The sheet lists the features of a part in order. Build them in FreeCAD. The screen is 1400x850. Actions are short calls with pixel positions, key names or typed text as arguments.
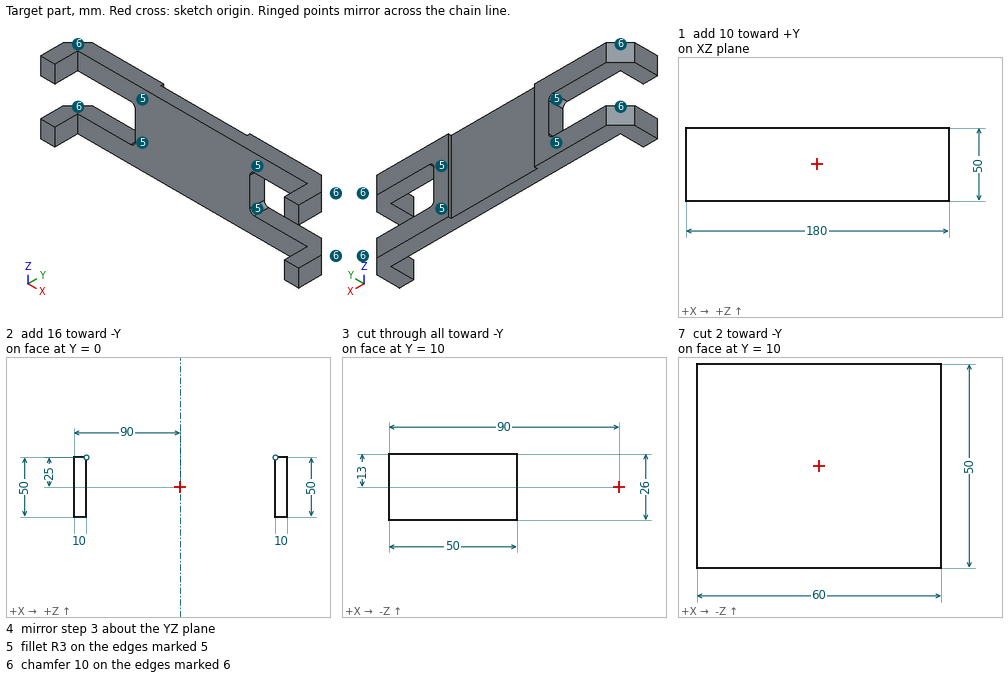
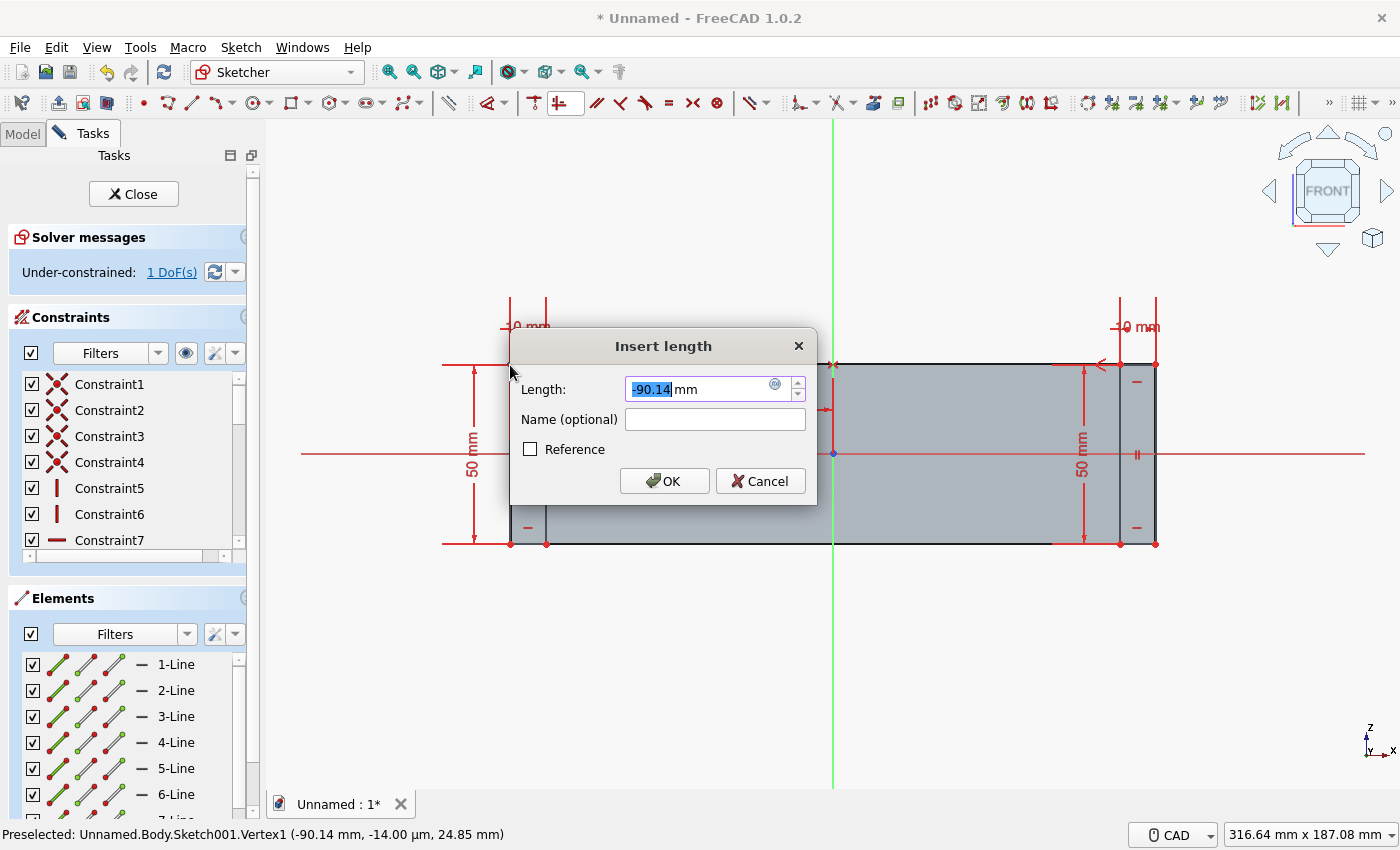
text(-90)
key(Return)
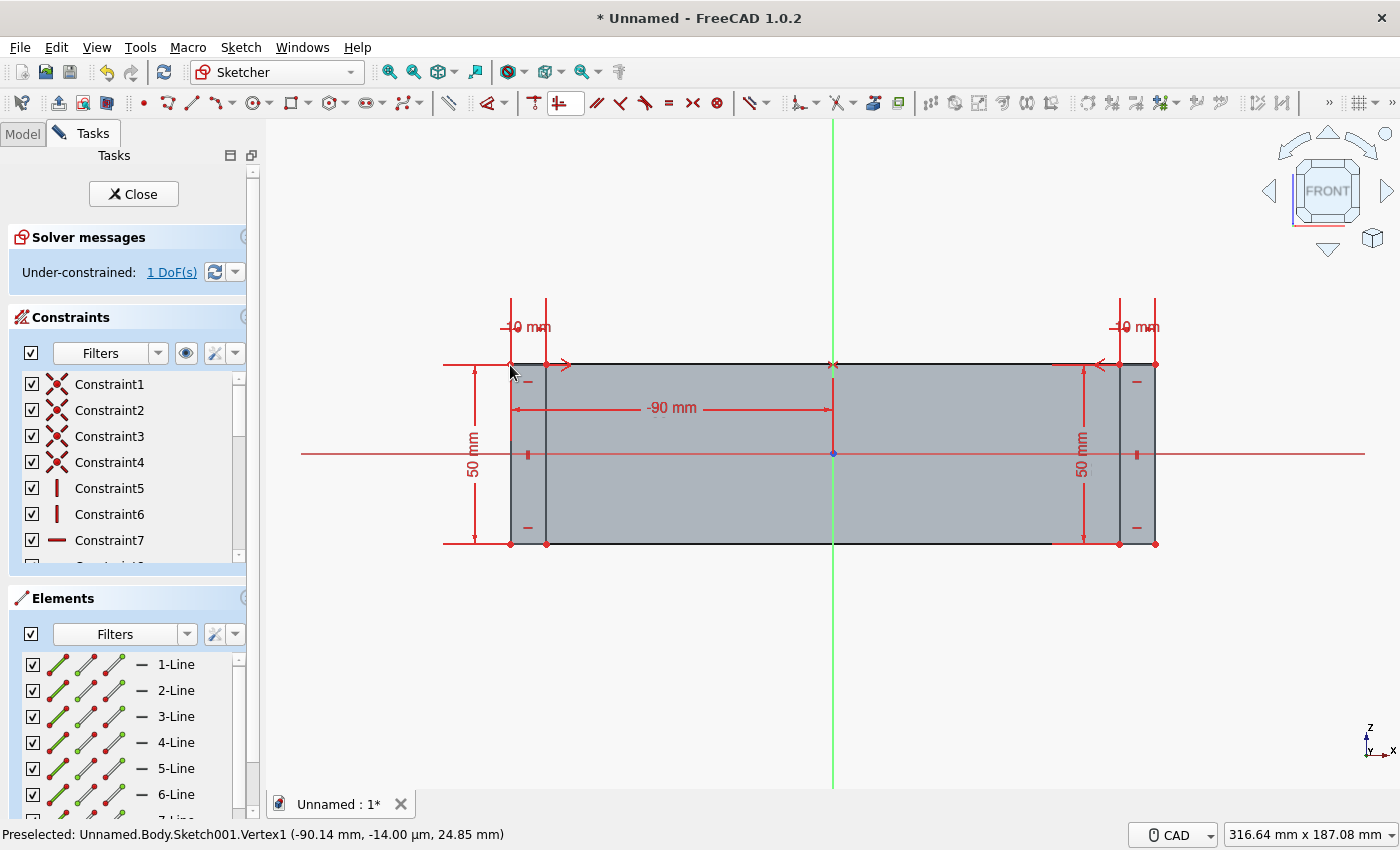
click(511, 365)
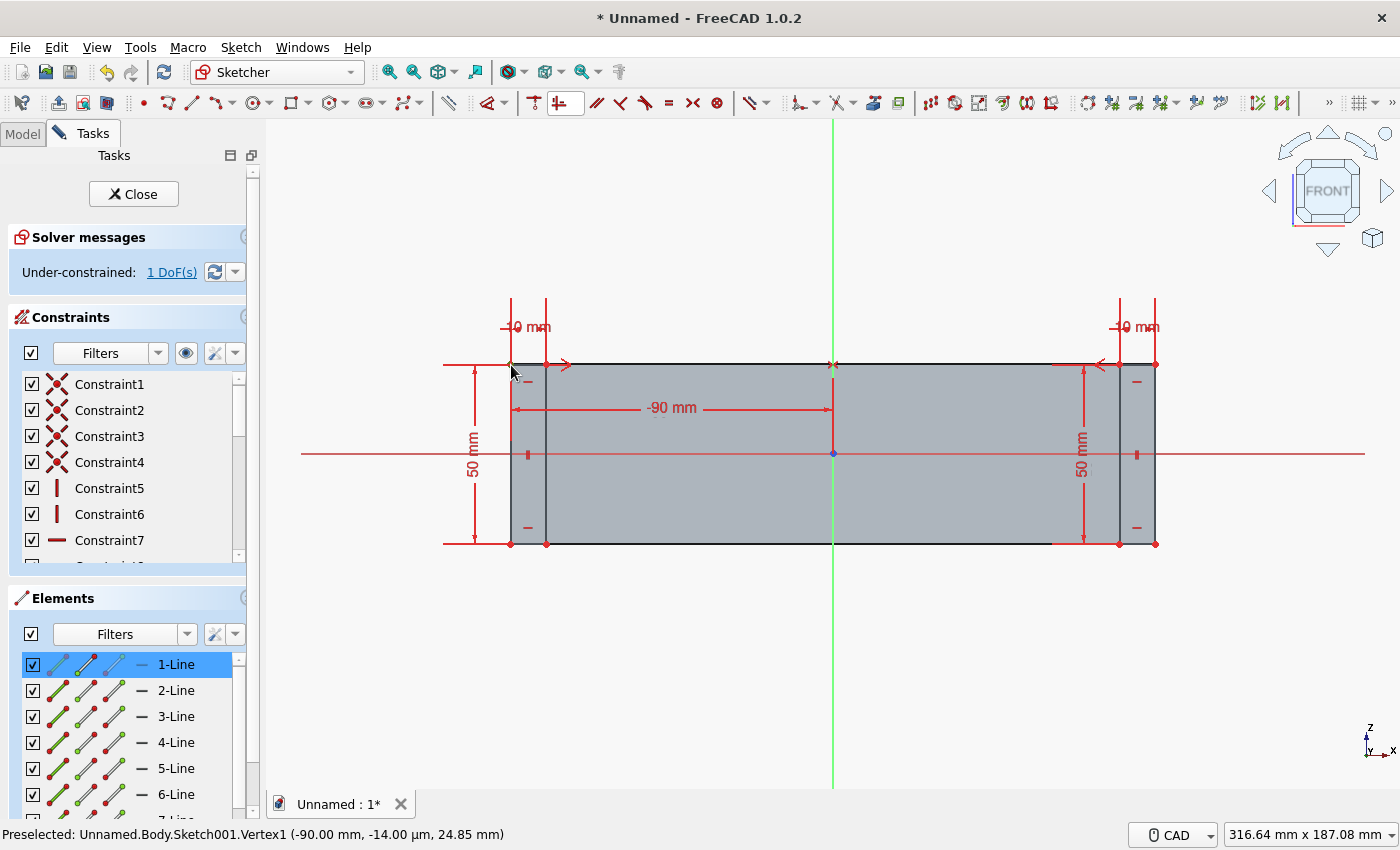
key(i)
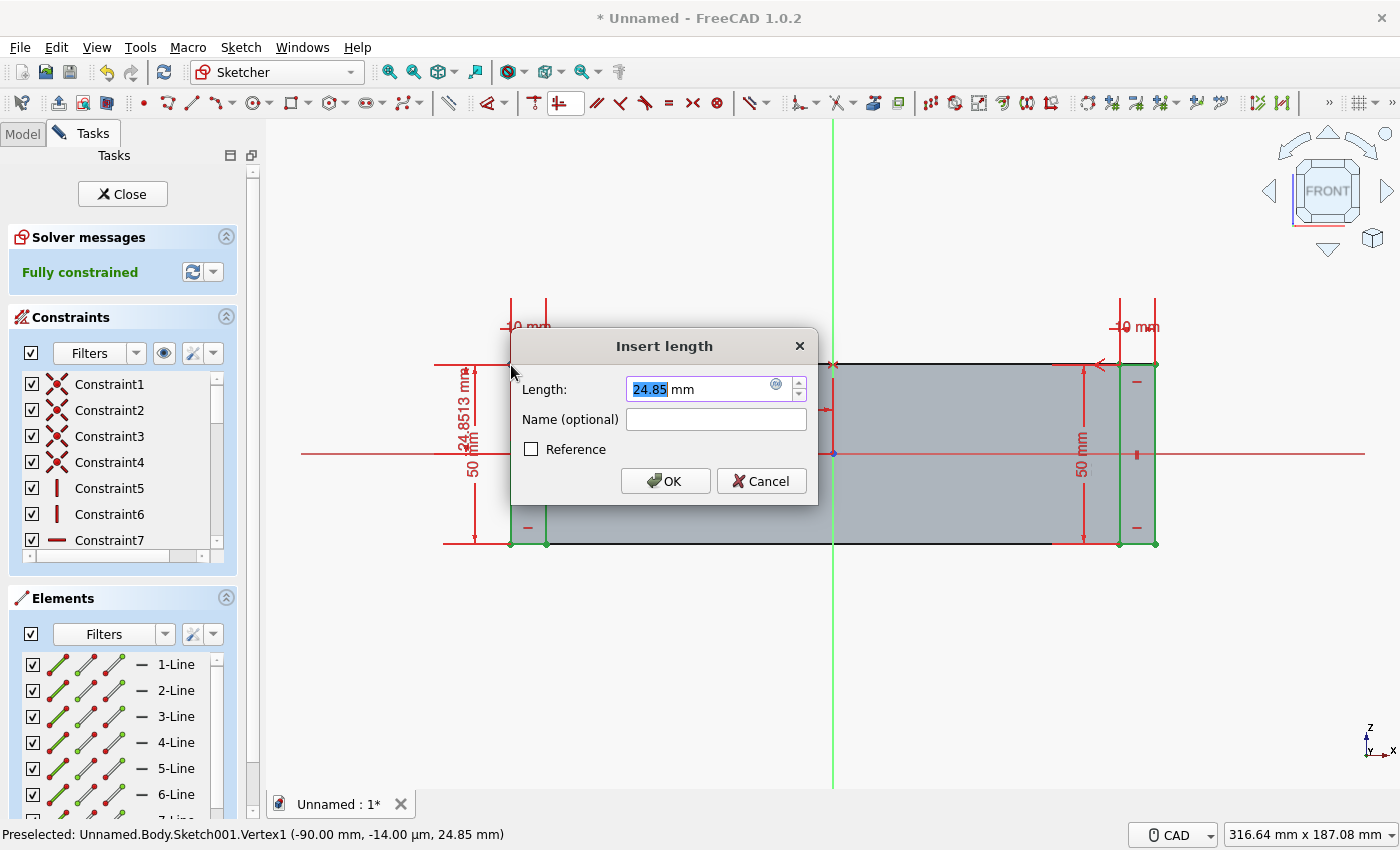
text(25)
key(Return)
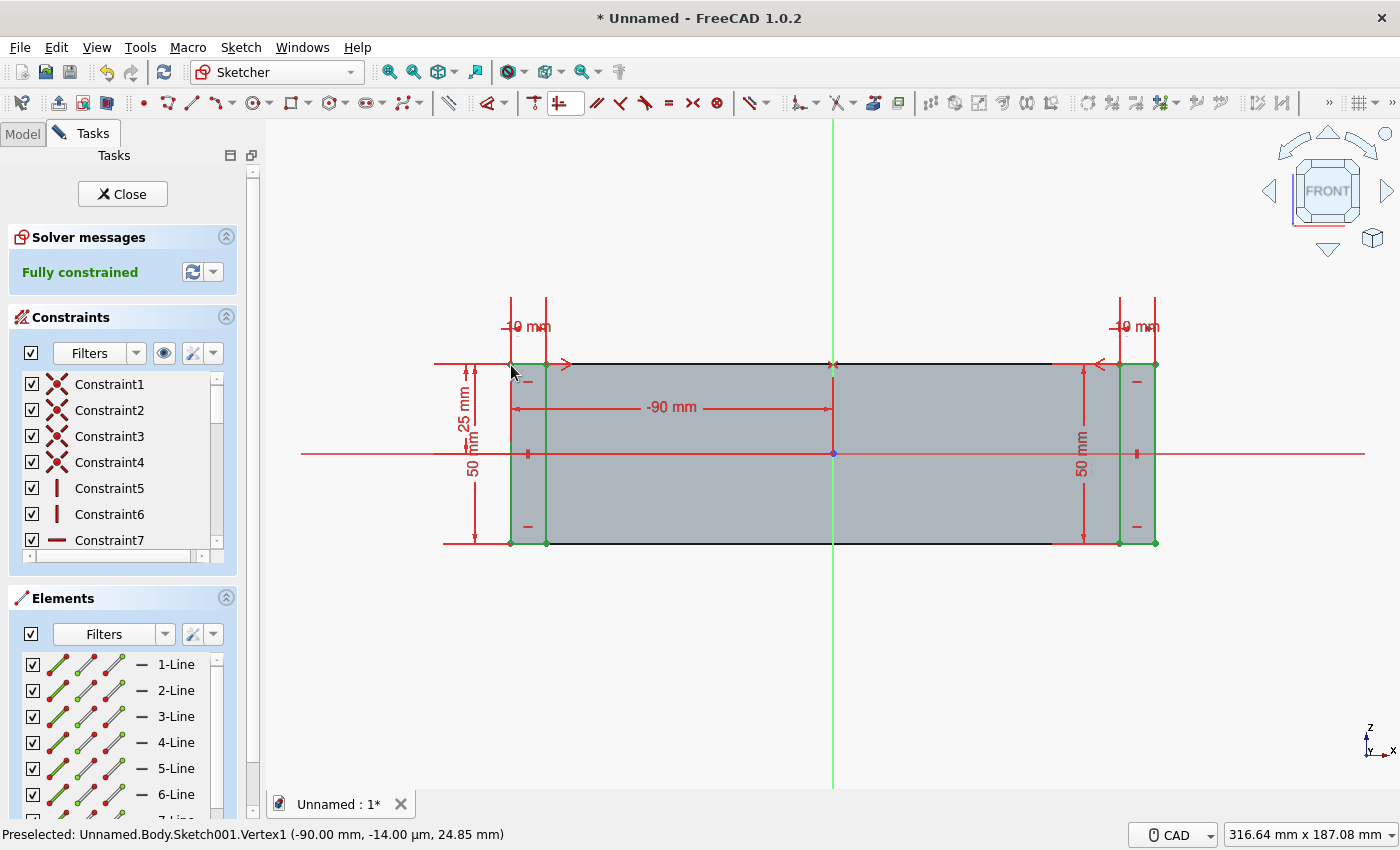
click(123, 194)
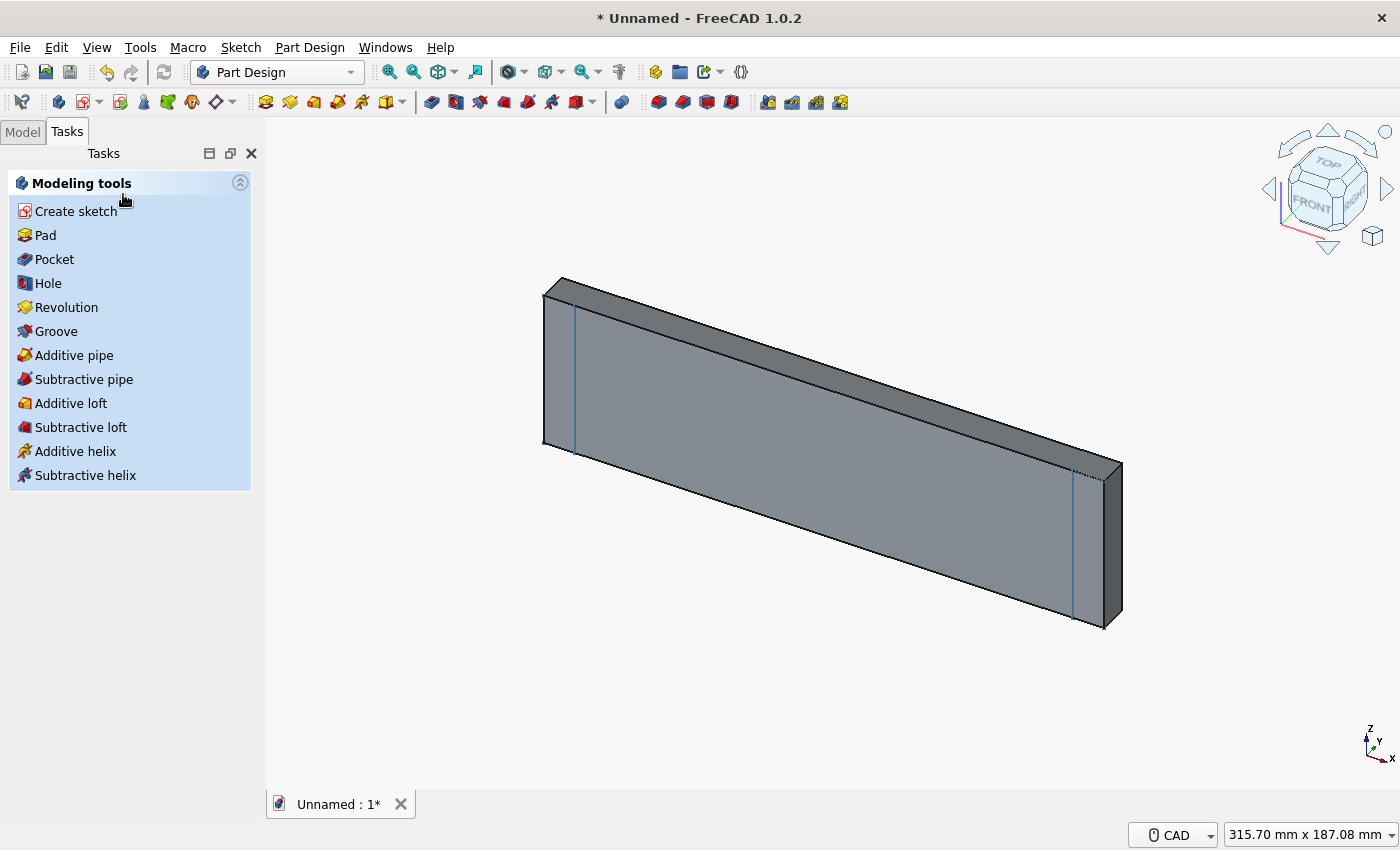
click(266, 102)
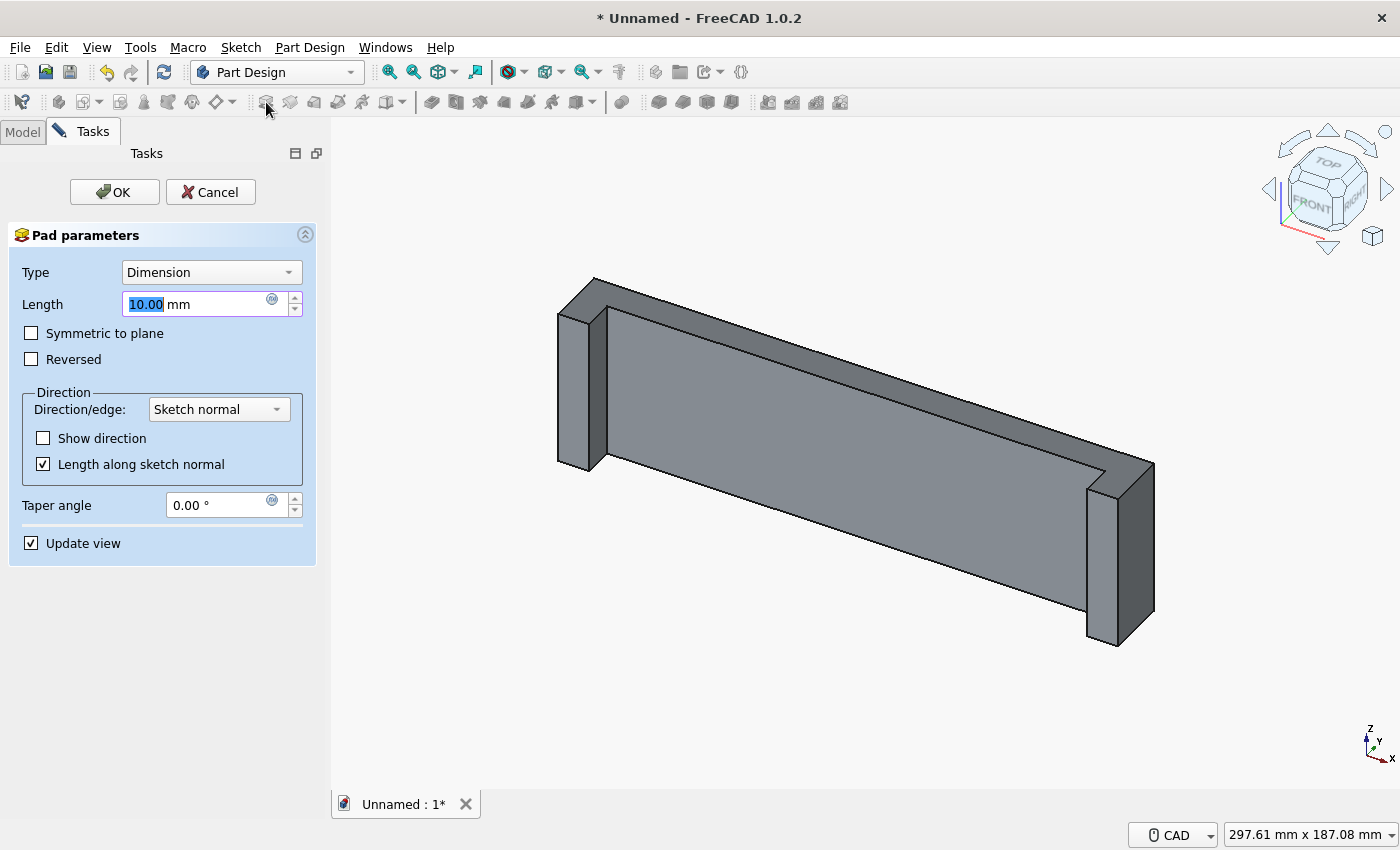
text(16)
key(Tab)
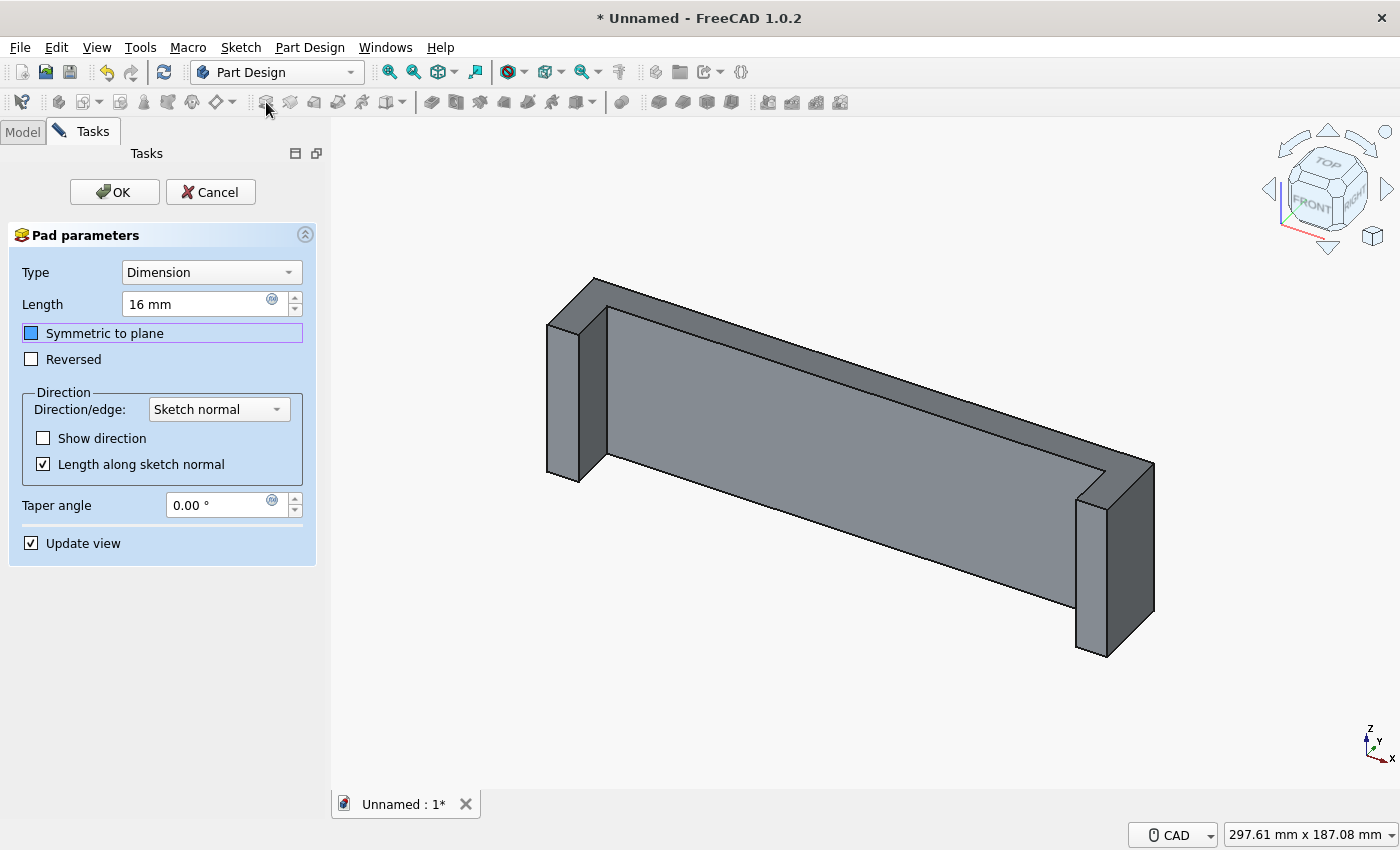
click(115, 192)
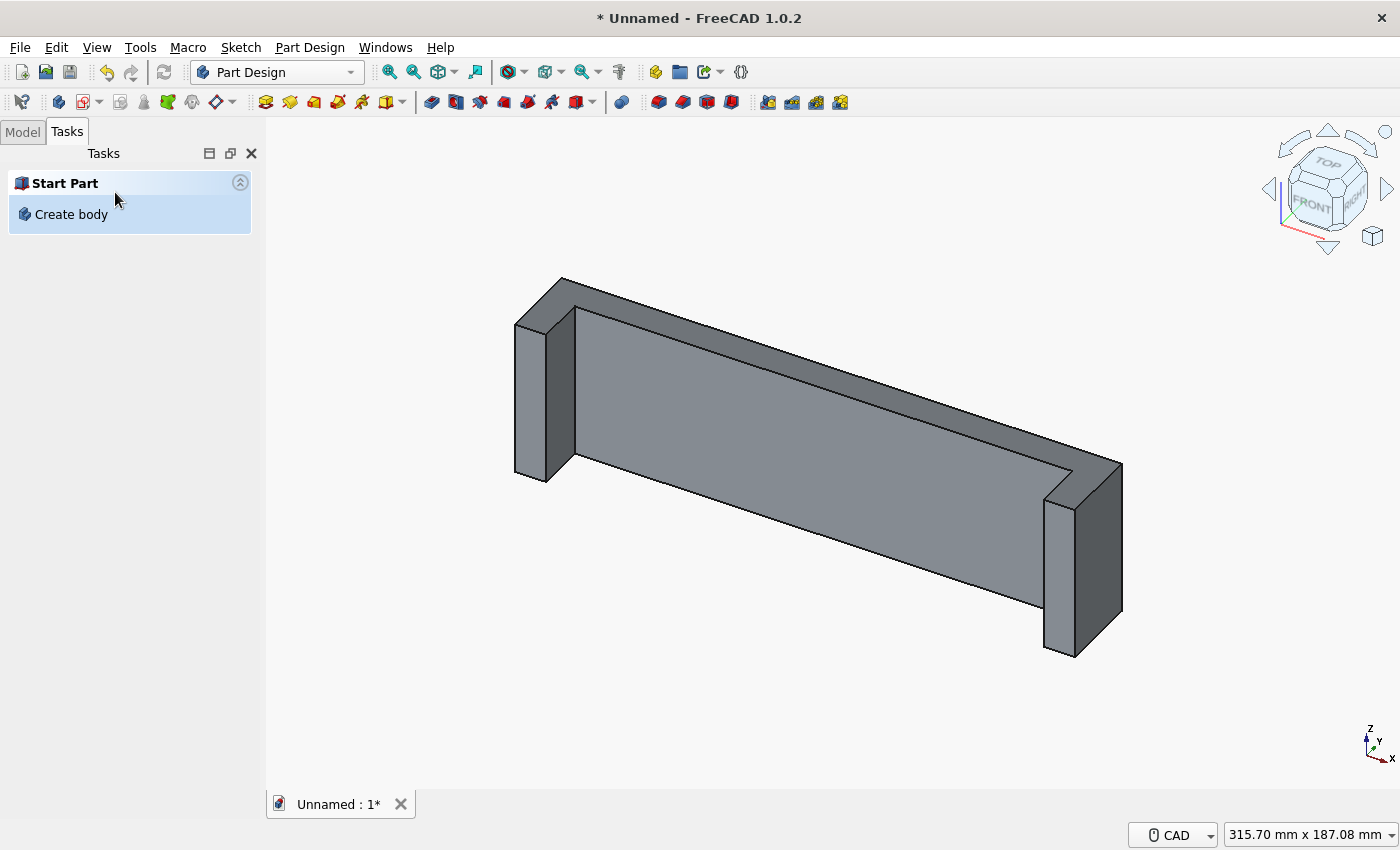
key(4)